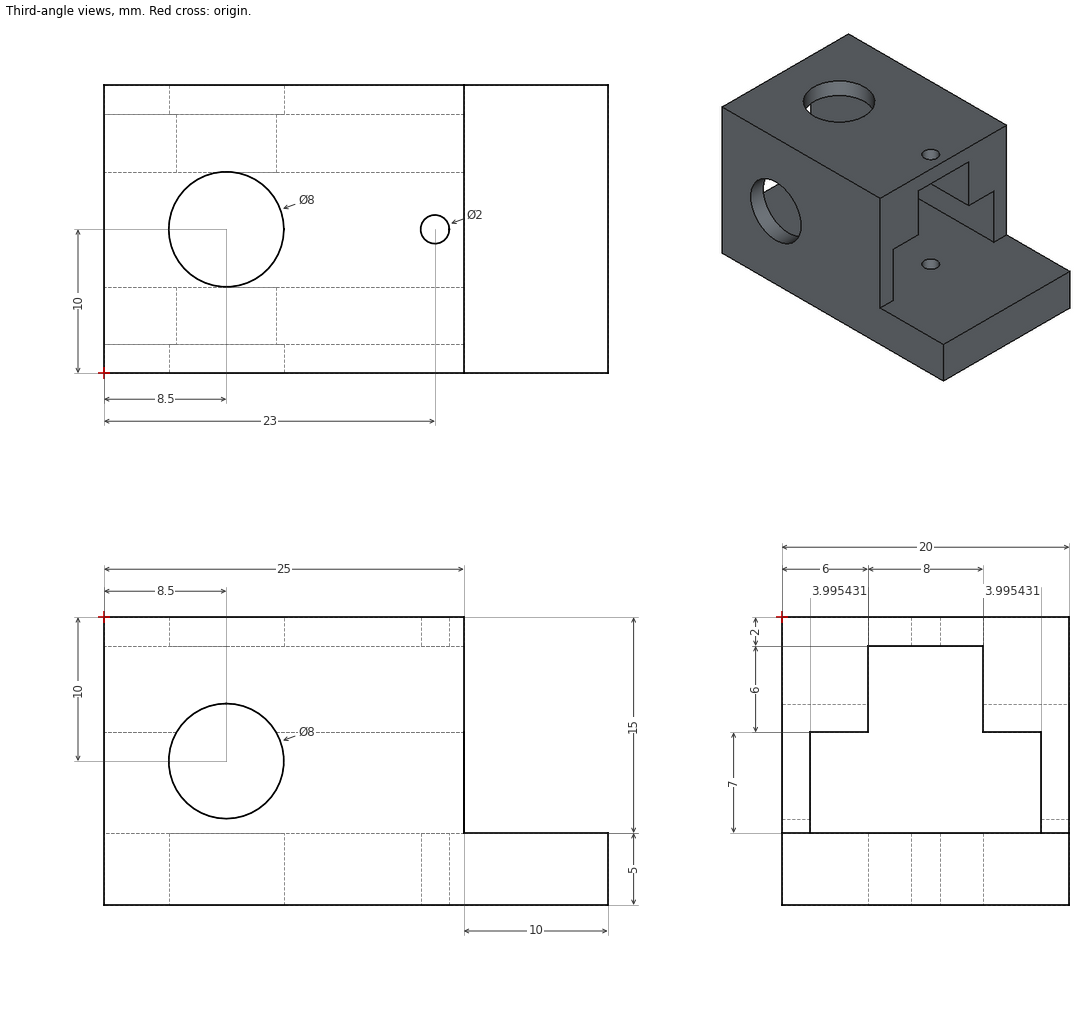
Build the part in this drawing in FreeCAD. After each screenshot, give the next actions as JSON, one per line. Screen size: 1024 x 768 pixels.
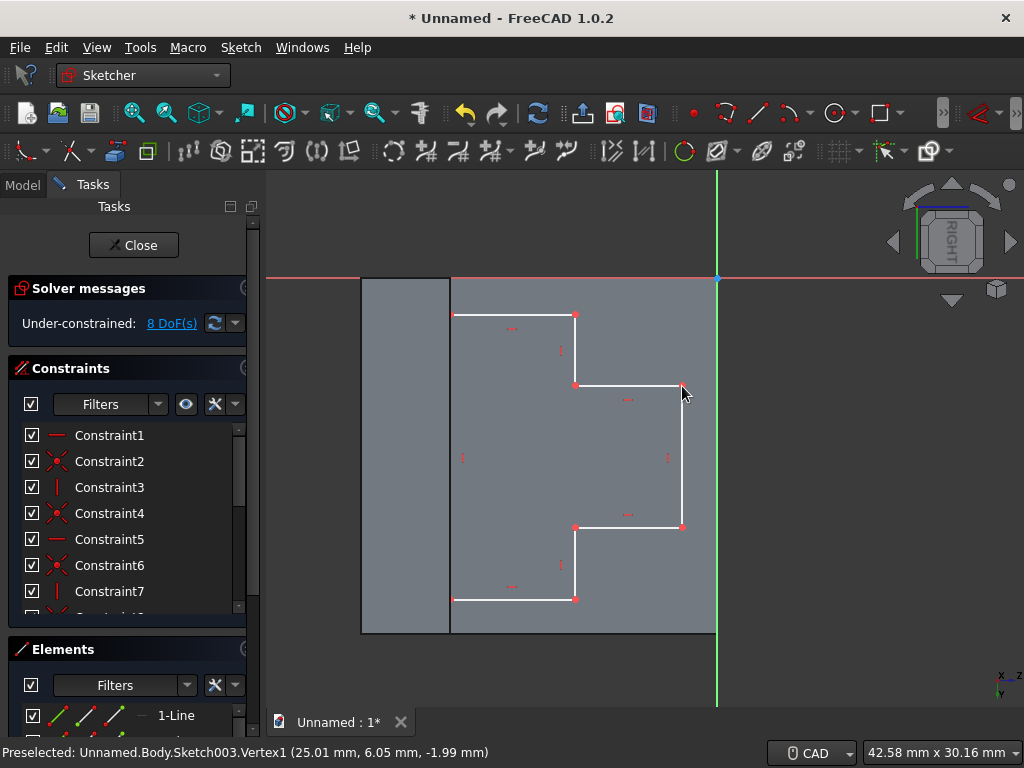
{"action": "left_click", "coordinate": [978, 114]}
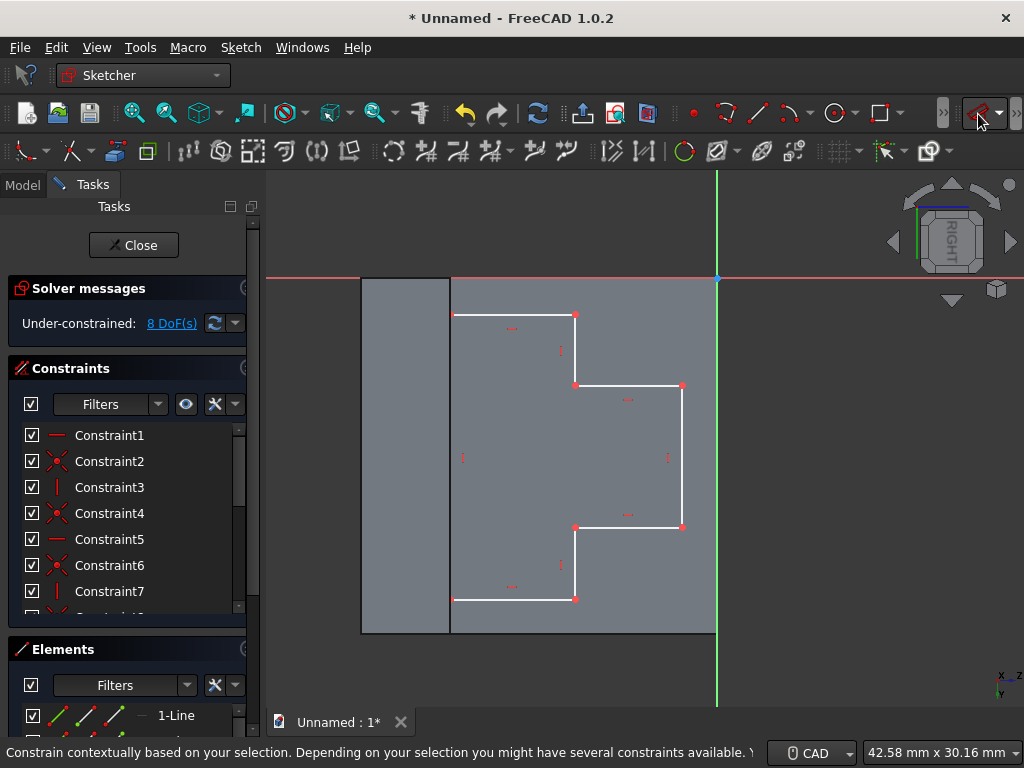
{"action": "left_click", "coordinate": [650, 386]}
{"action": "left_click", "coordinate": [629, 352]}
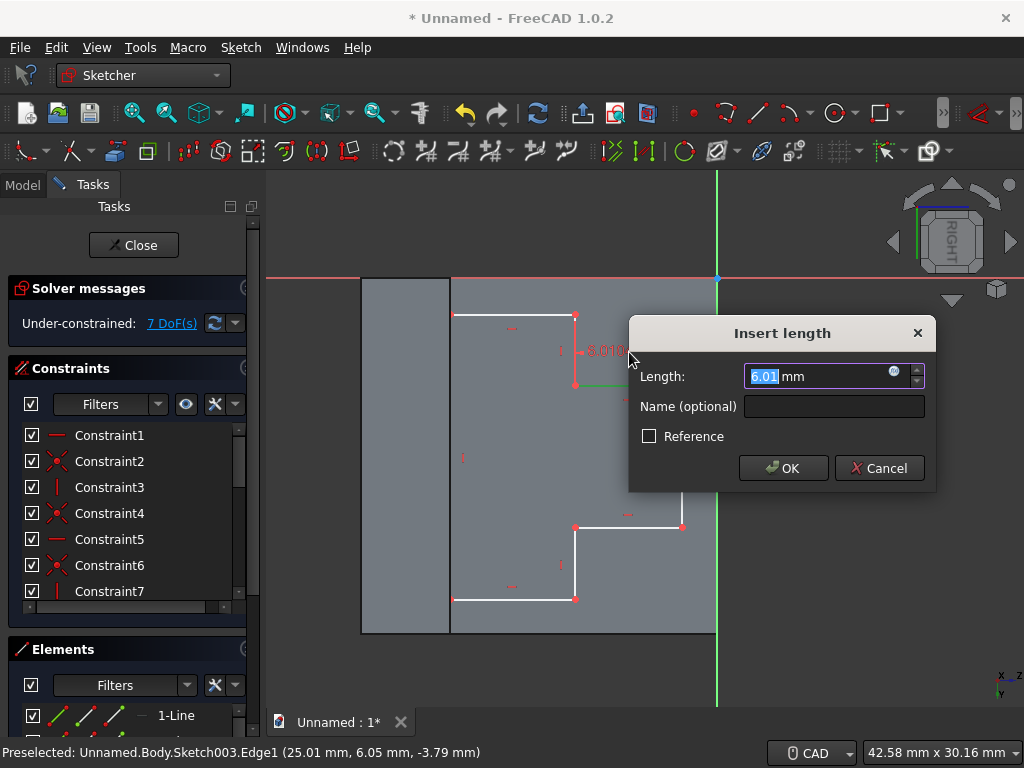
{"action": "type", "text": "6"}
{"action": "key", "text": "Return"}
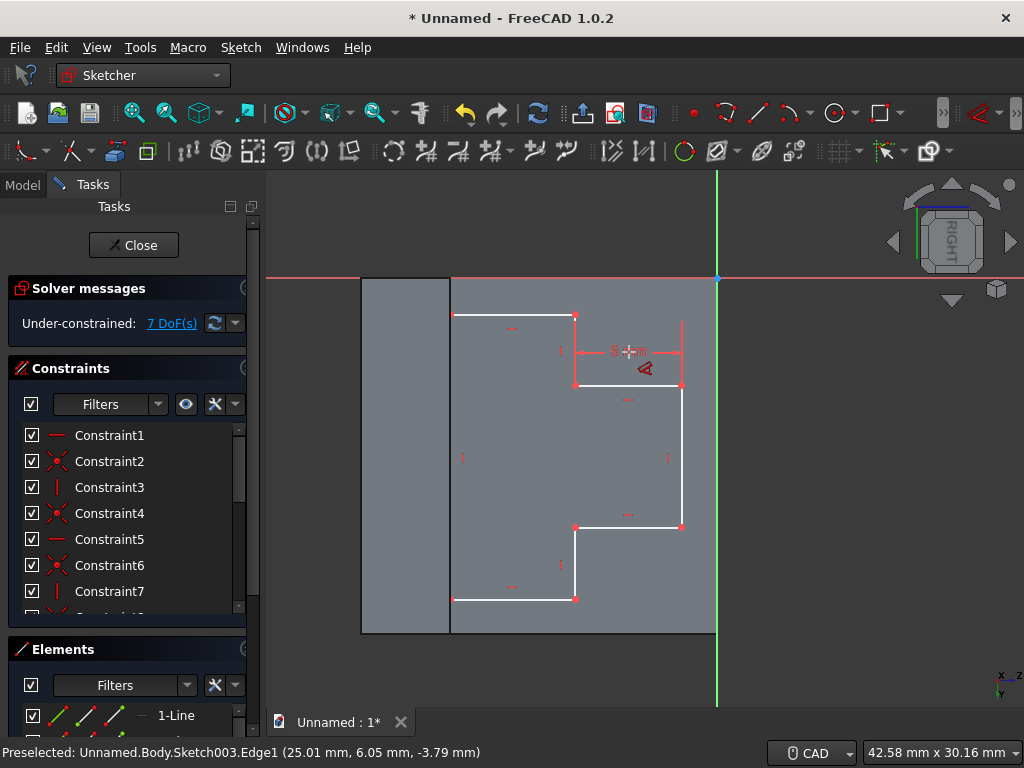
{"action": "left_click", "coordinate": [538, 315]}
{"action": "left_click", "coordinate": [513, 349]}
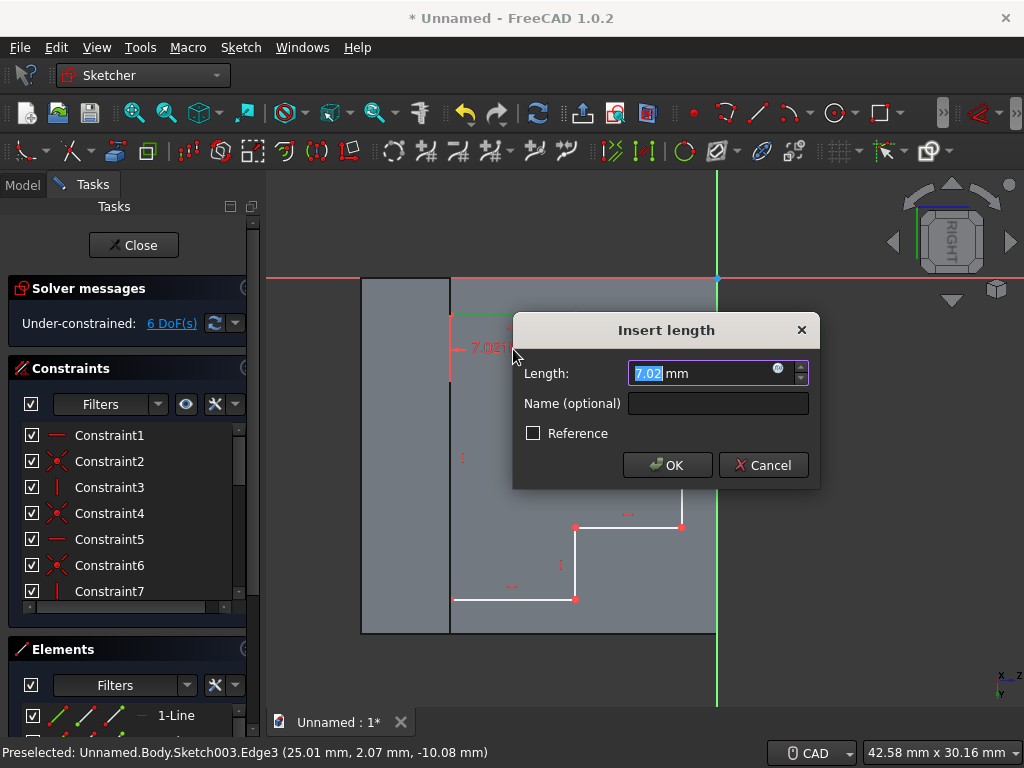
{"action": "type", "text": "7"}
{"action": "key", "text": "Return"}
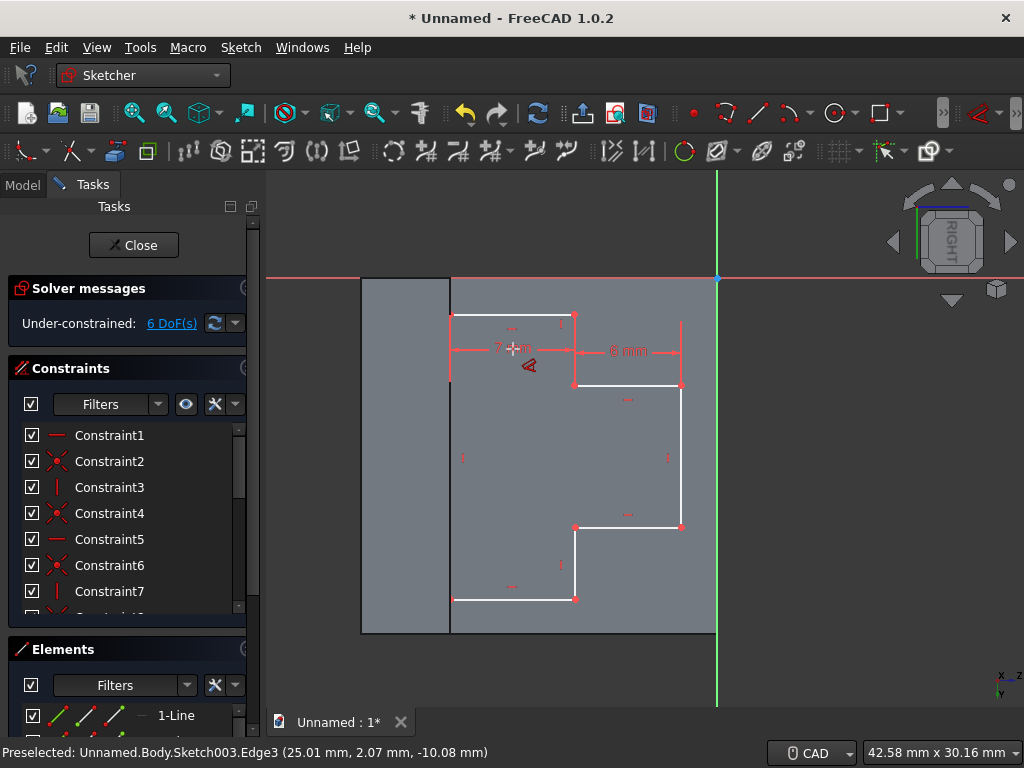
{"action": "left_click", "coordinate": [487, 600]}
{"action": "left_click", "coordinate": [513, 634]}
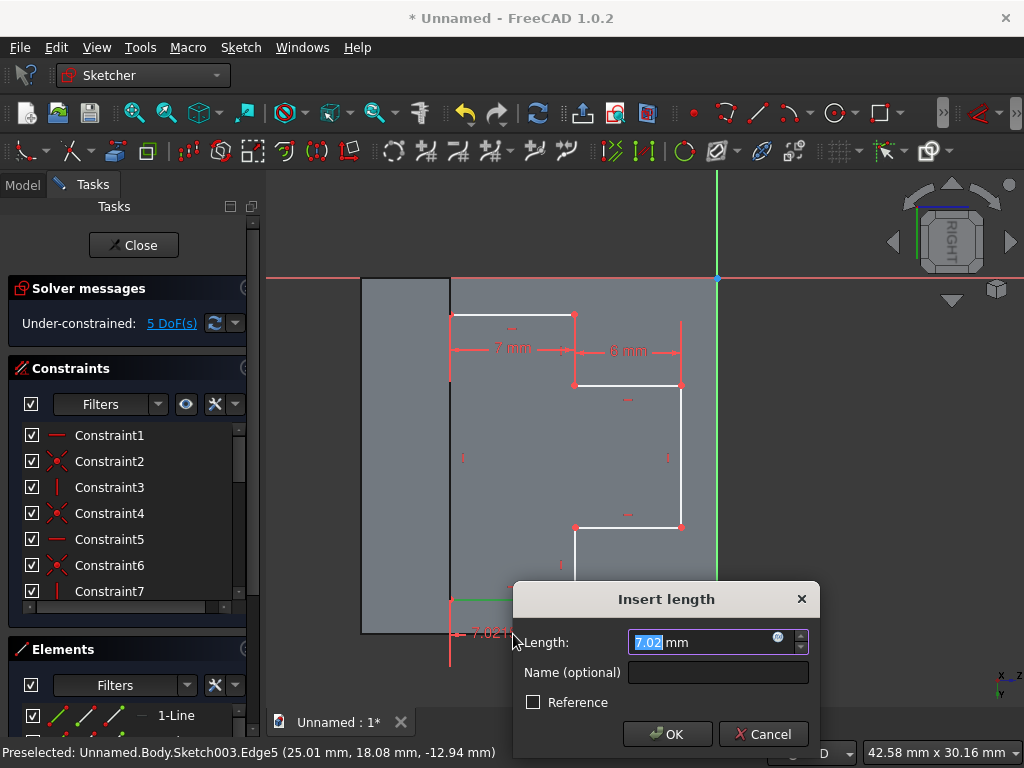
{"action": "type", "text": "7"}
{"action": "key", "text": "Return"}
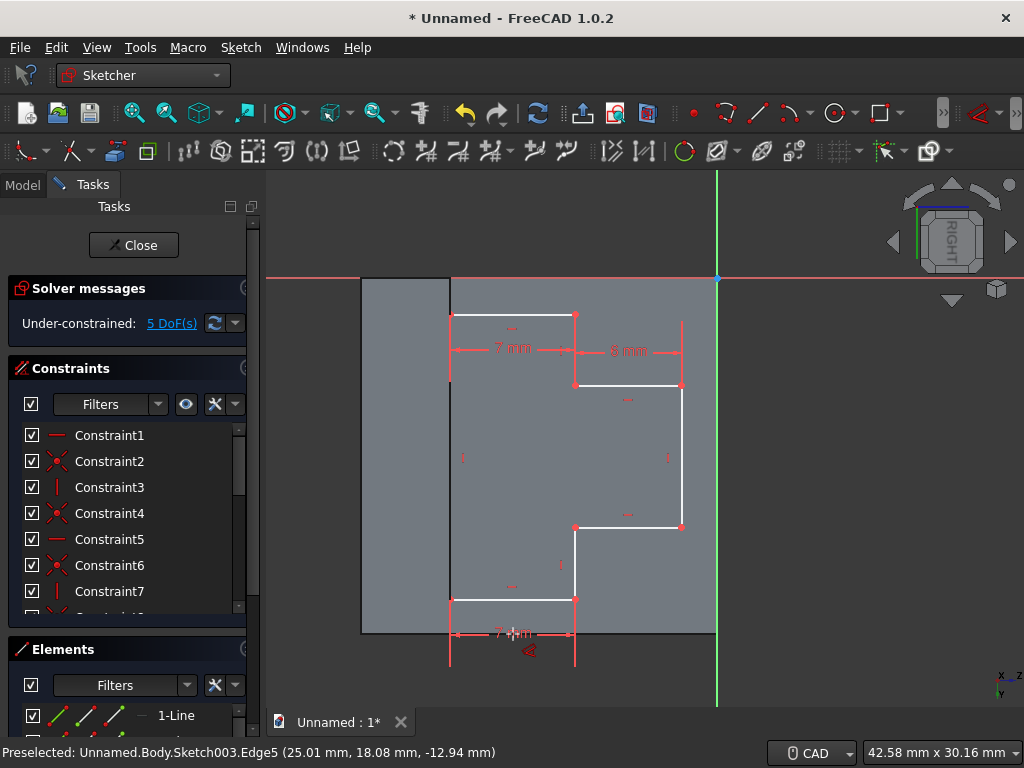
{"action": "left_click", "coordinate": [682, 485]}
{"action": "left_click", "coordinate": [648, 457]}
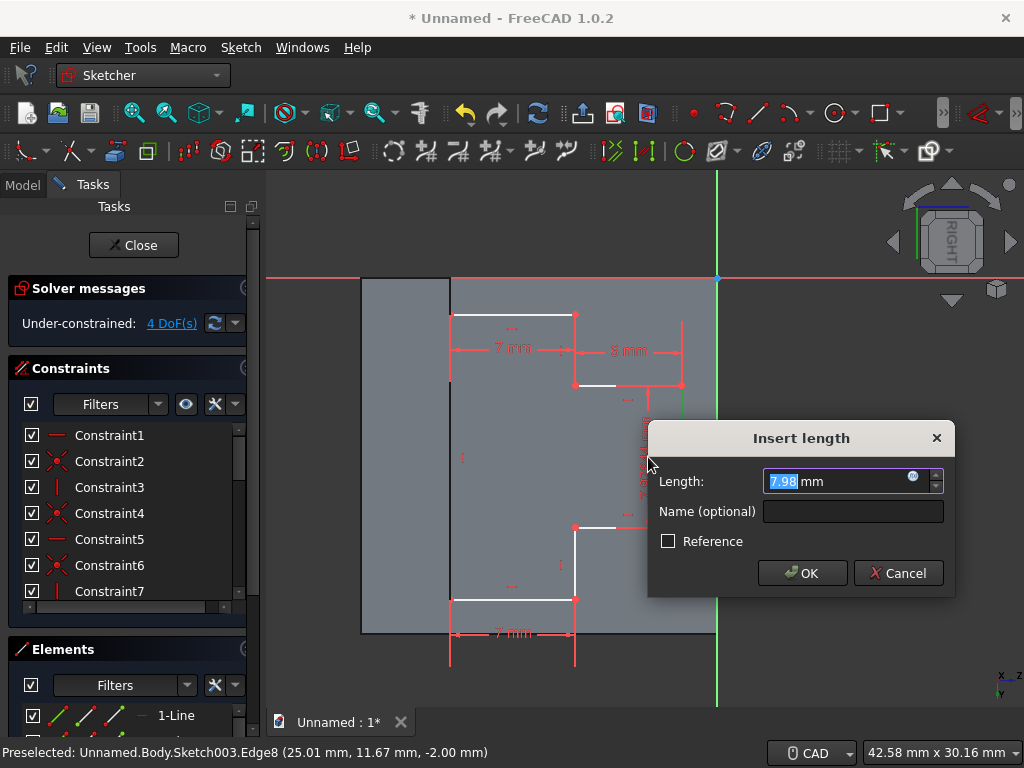
{"action": "type", "text": "8"}
{"action": "key", "text": "Return"}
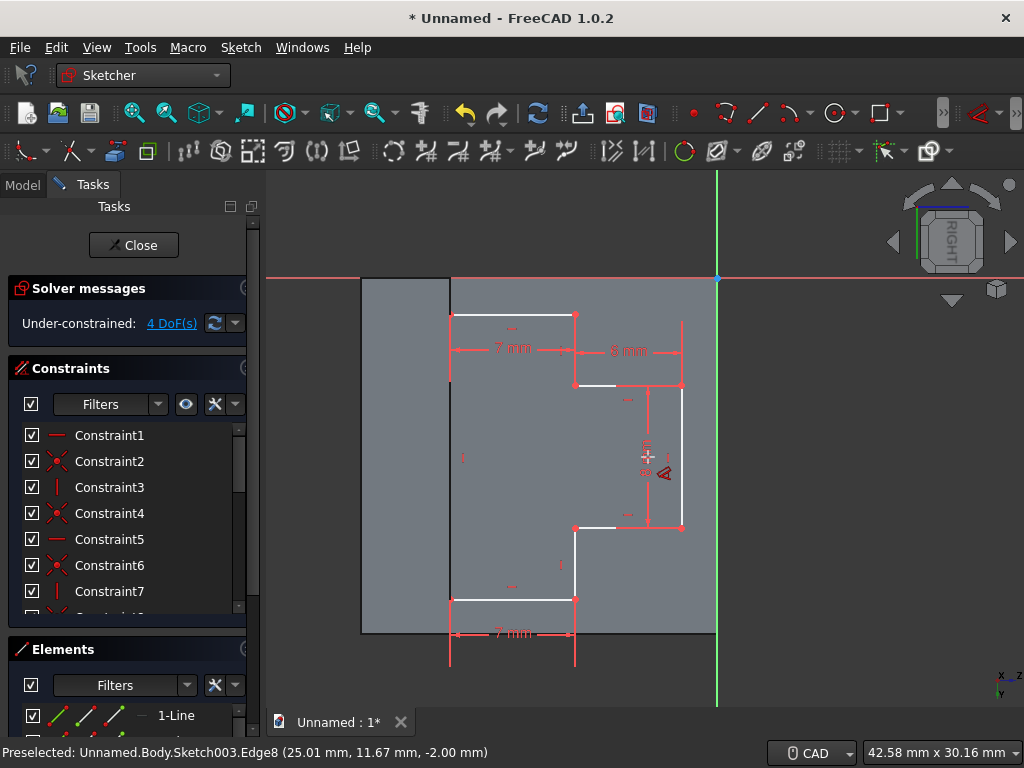
{"action": "left_click", "coordinate": [682, 386]}
{"action": "left_click", "coordinate": [700, 244]}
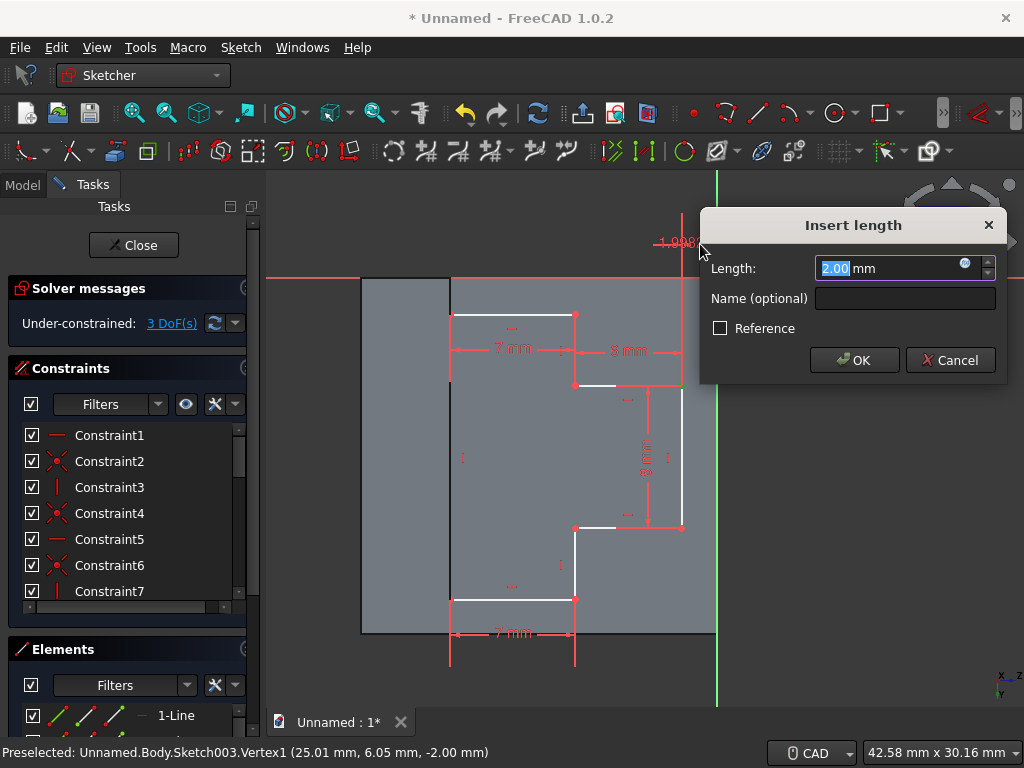
{"action": "type", "text": "2"}
{"action": "key", "text": "Return"}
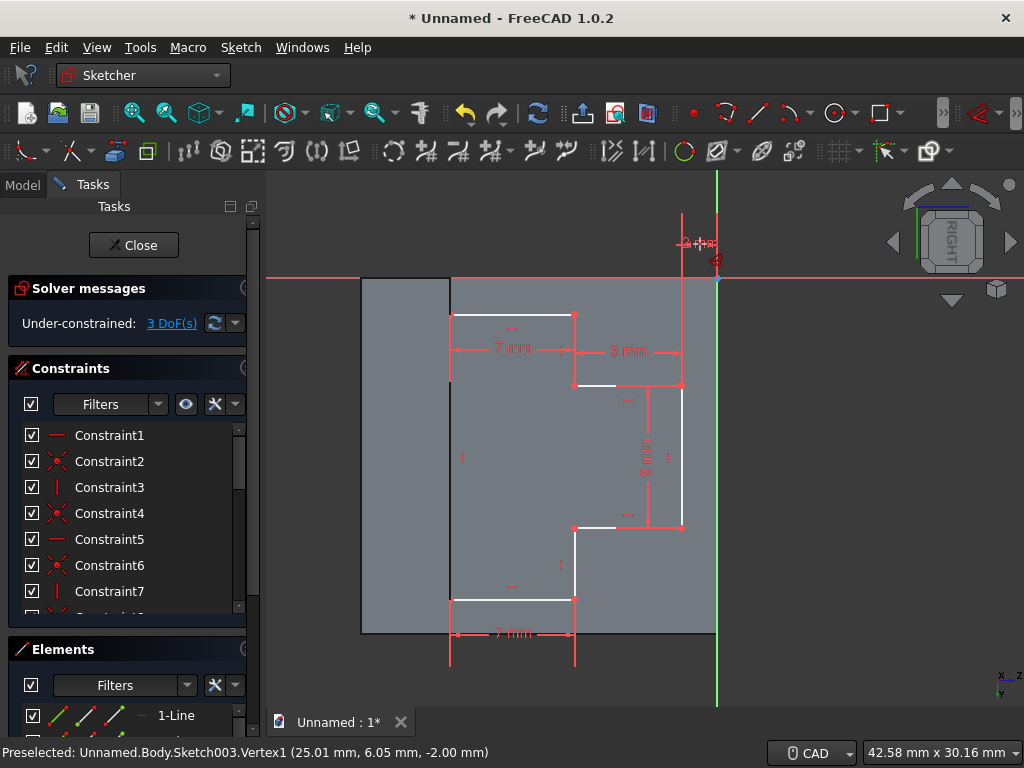
{"action": "left_click", "coordinate": [682, 386]}
{"action": "left_click", "coordinate": [751, 332]}